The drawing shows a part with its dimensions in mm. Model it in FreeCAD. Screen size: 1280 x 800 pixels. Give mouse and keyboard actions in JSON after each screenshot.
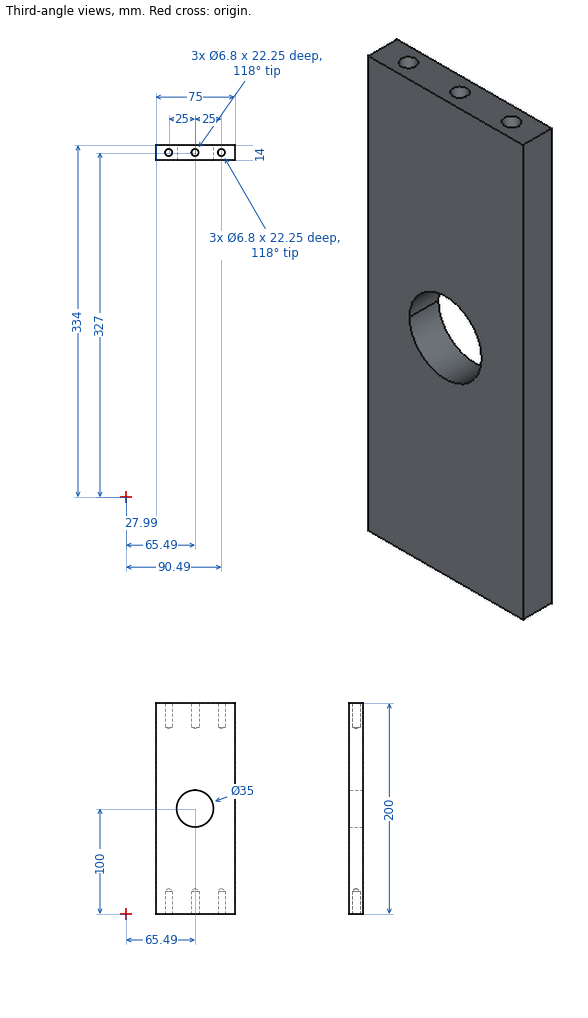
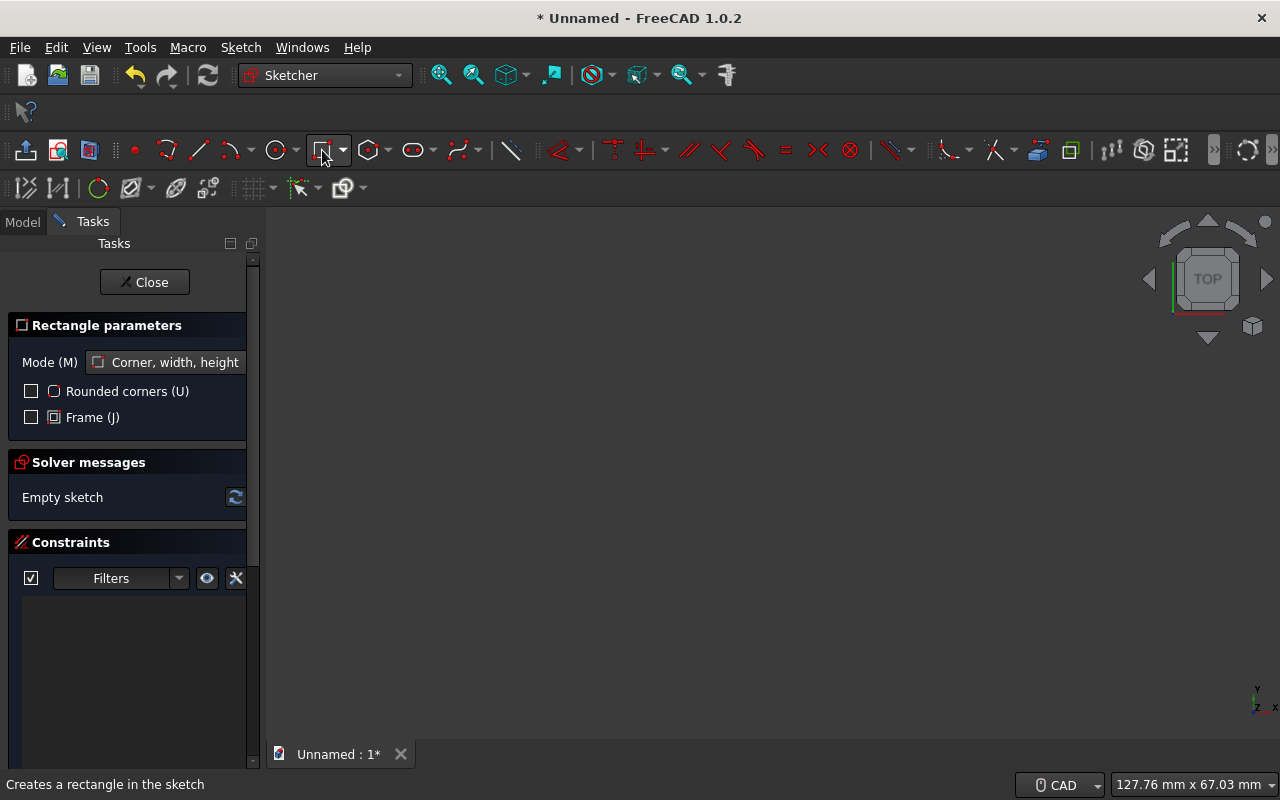
{"action": "left_click", "coordinate": [407, 417]}
{"action": "mouse_move", "coordinate": [1002, 528]}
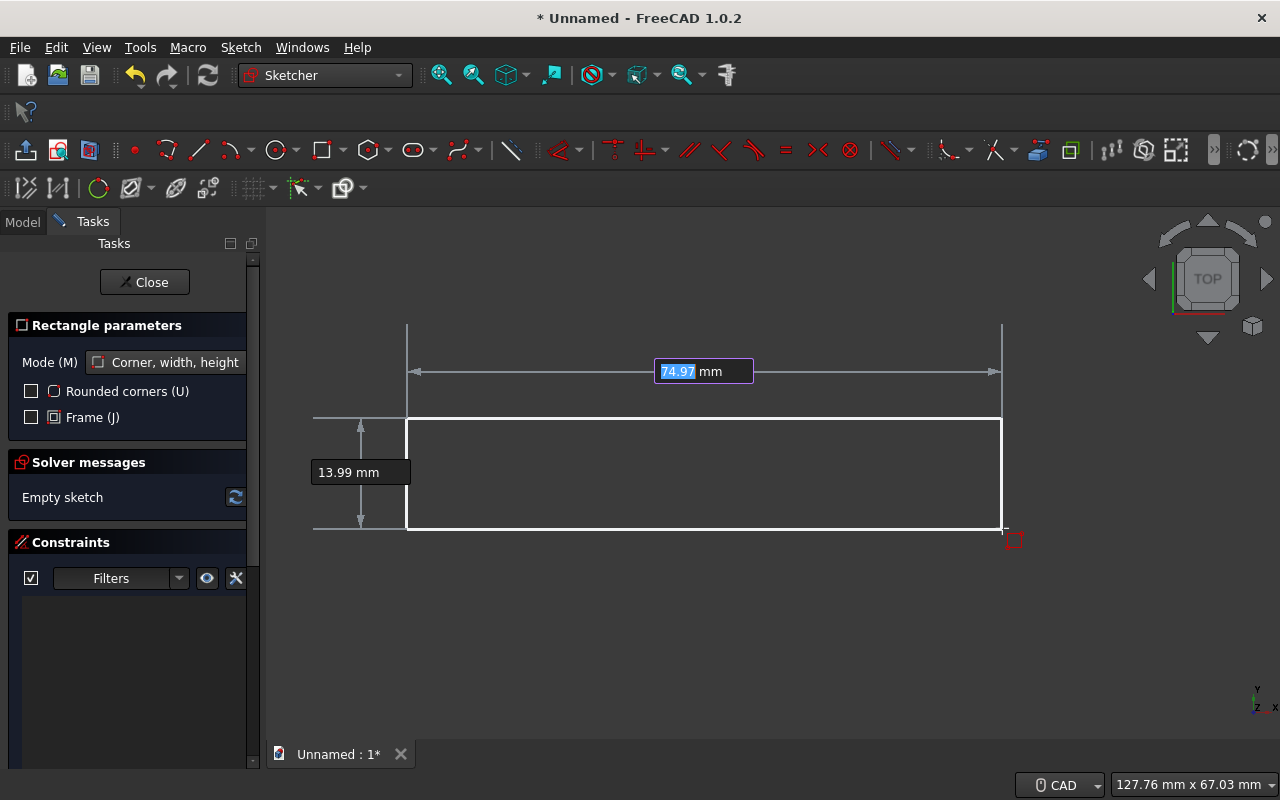
{"action": "type", "text": "75"}
{"action": "key", "text": "Tab"}
{"action": "type", "text": "14"}
{"action": "key", "text": "Return"}
{"action": "key", "text": "Escape"}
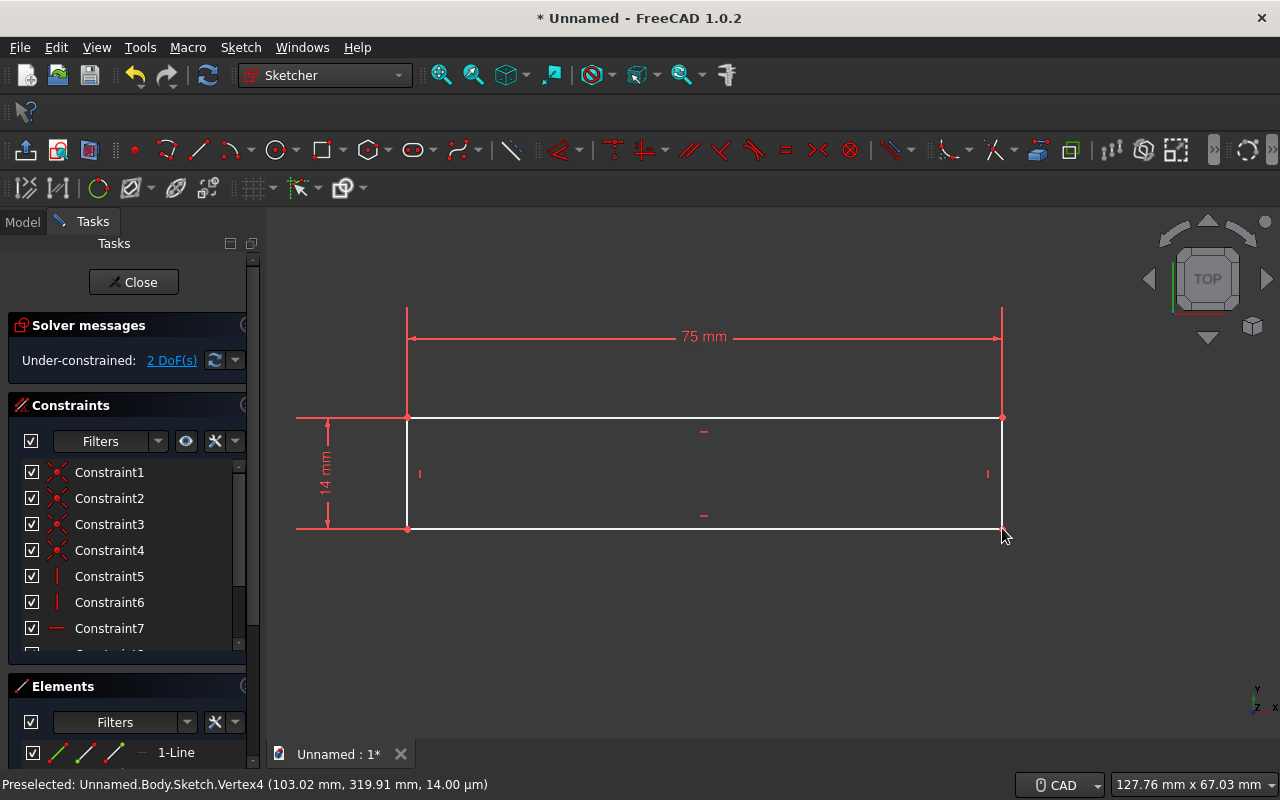
{"action": "left_click", "coordinate": [407, 418]}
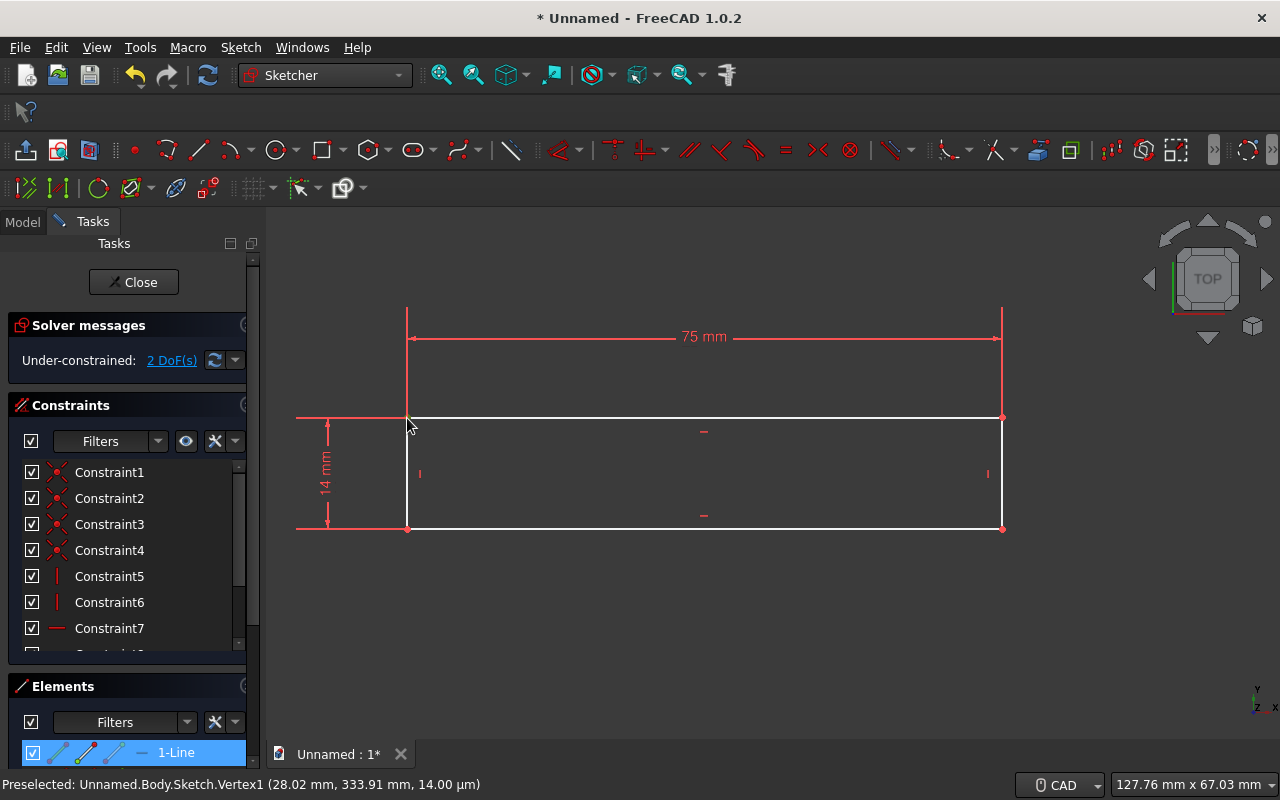
{"action": "left_click", "coordinate": [582, 150]}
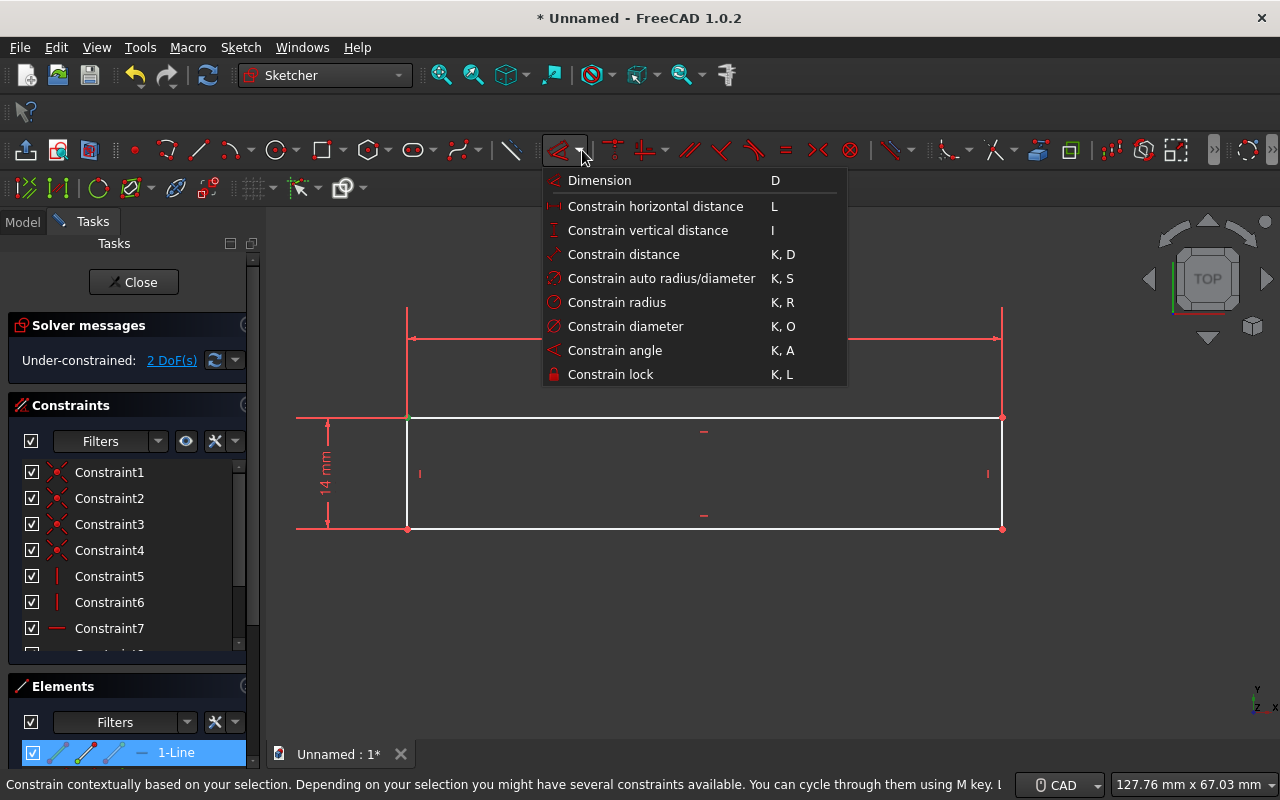
{"action": "left_click", "coordinate": [695, 230]}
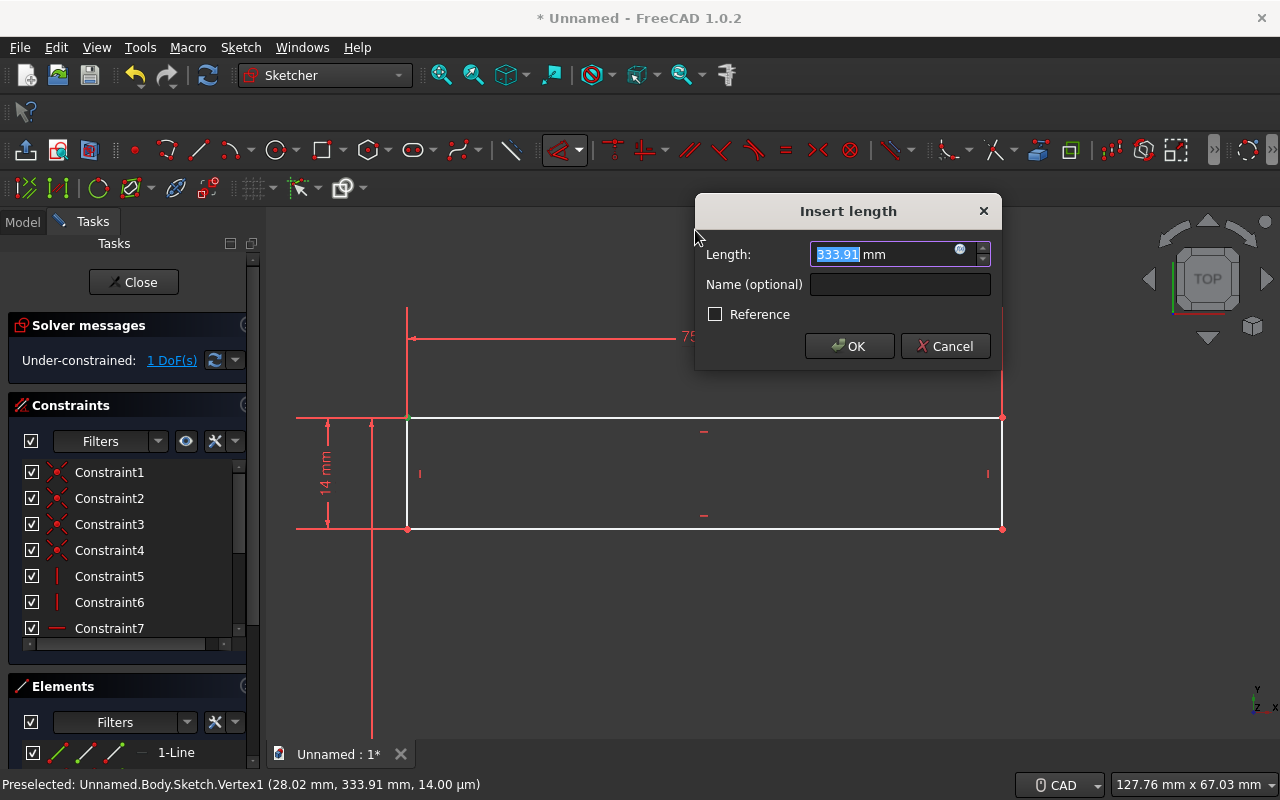
{"action": "type", "text": "334"}
{"action": "key", "text": "Return"}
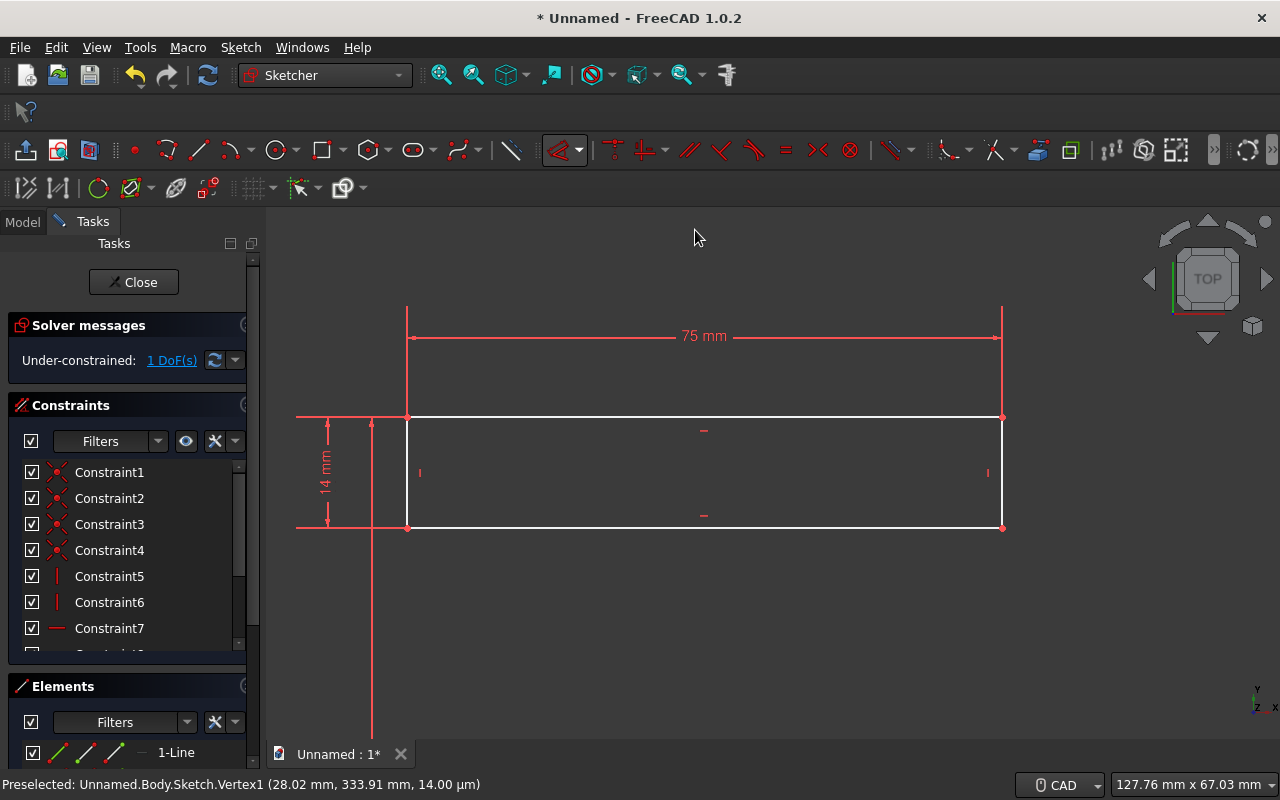
{"action": "left_click", "coordinate": [407, 417]}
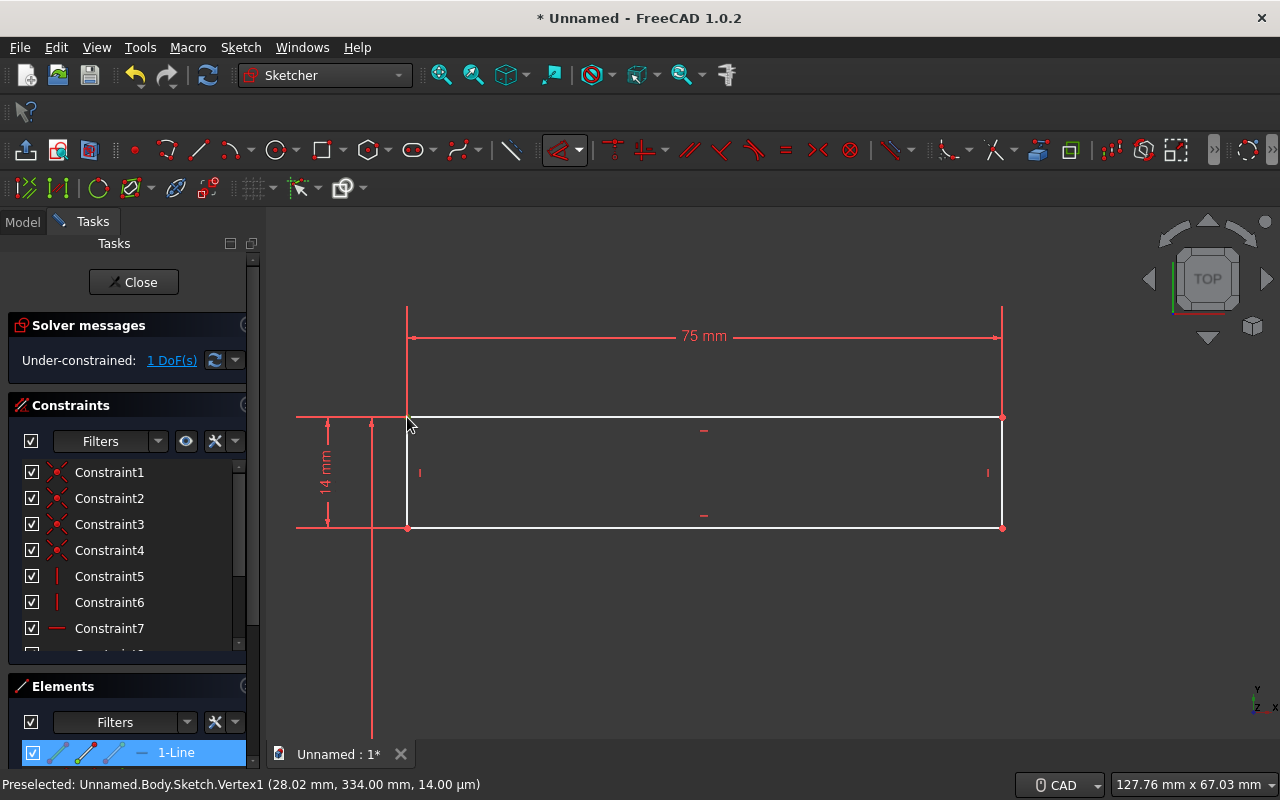
{"action": "left_click", "coordinate": [582, 150]}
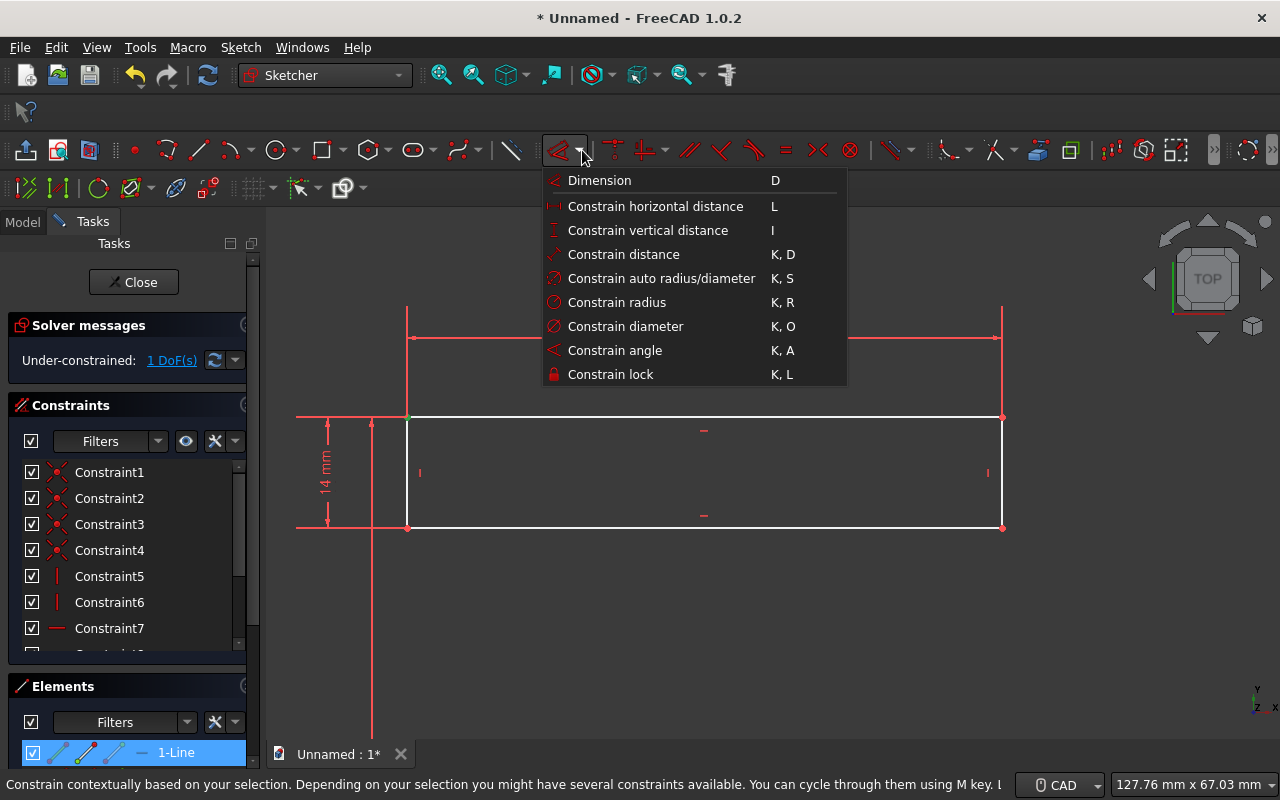
{"action": "left_click", "coordinate": [695, 206]}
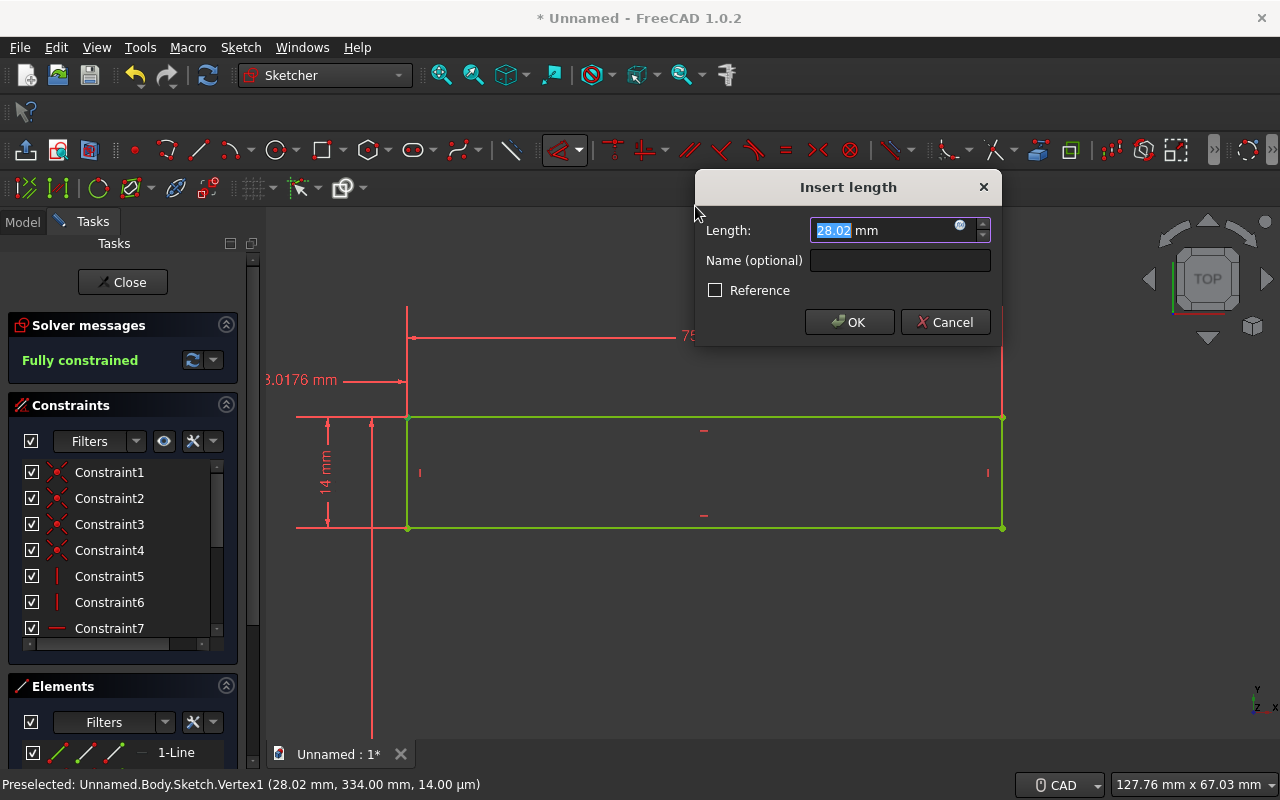
{"action": "type", "text": "27.99"}
{"action": "key", "text": "Return"}